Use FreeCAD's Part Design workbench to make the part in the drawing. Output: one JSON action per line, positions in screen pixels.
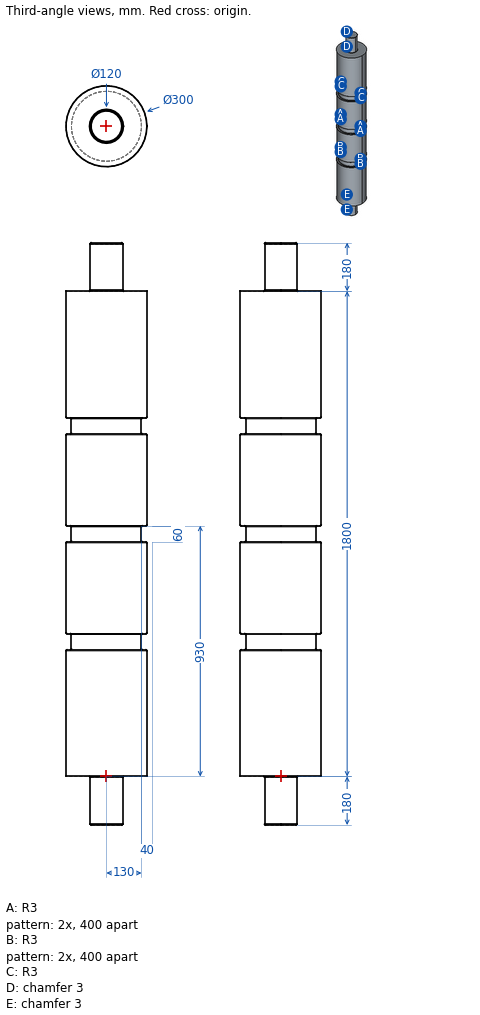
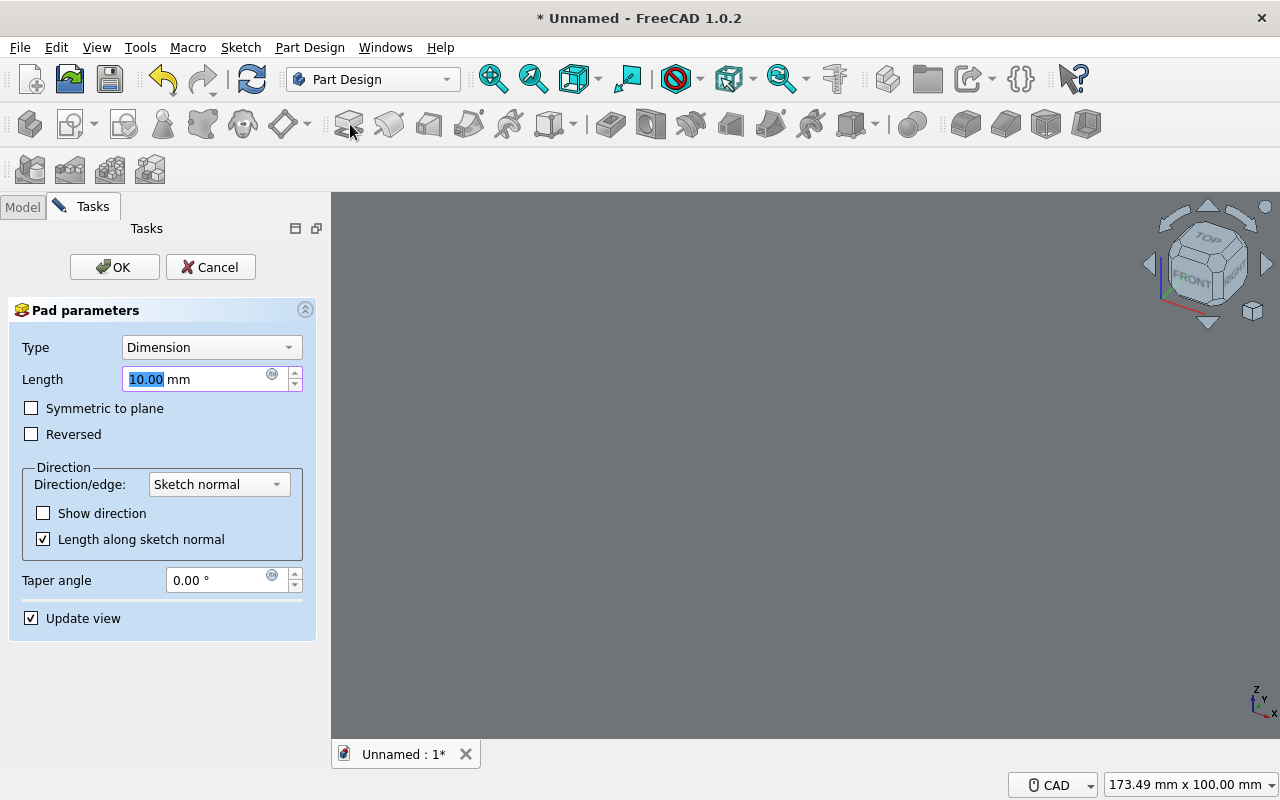
{"action": "type", "text": "1800"}
{"action": "key", "text": "Tab"}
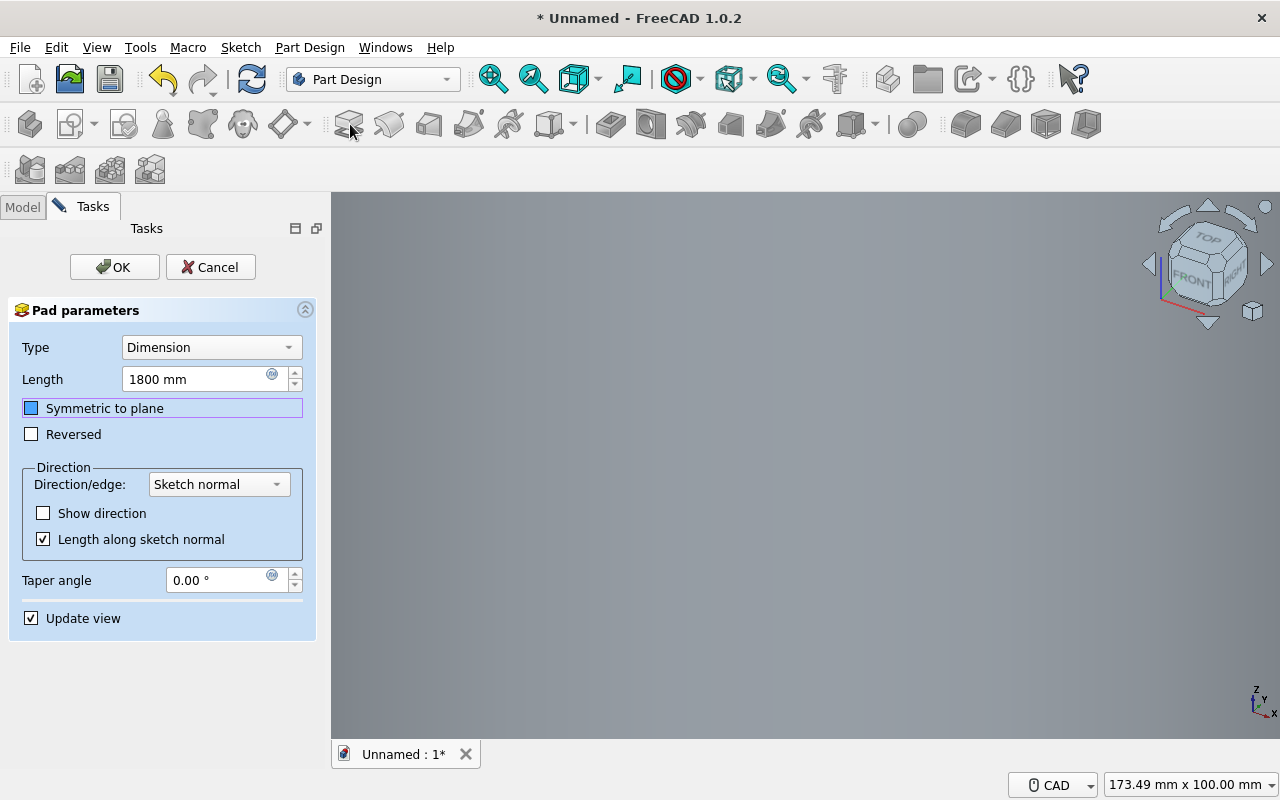
{"action": "left_click", "coordinate": [115, 267]}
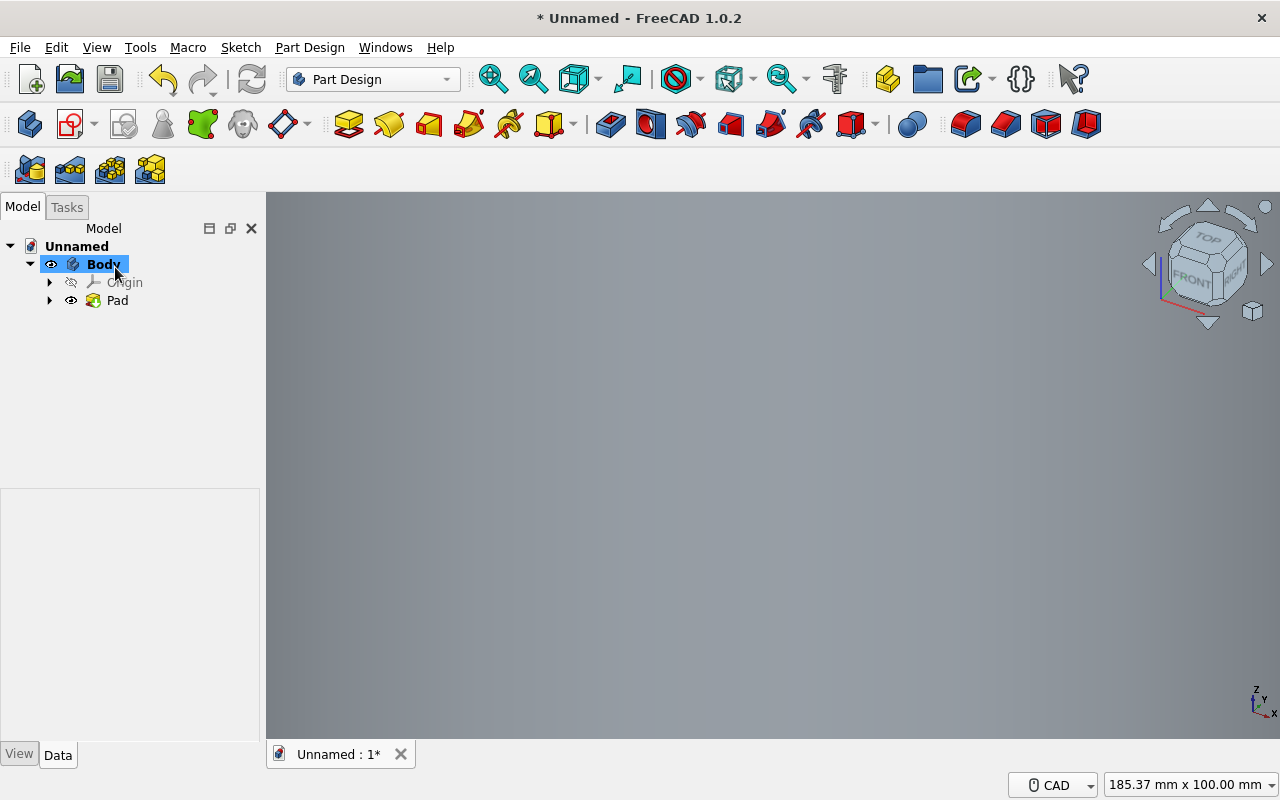
{"action": "left_click", "coordinate": [494, 80]}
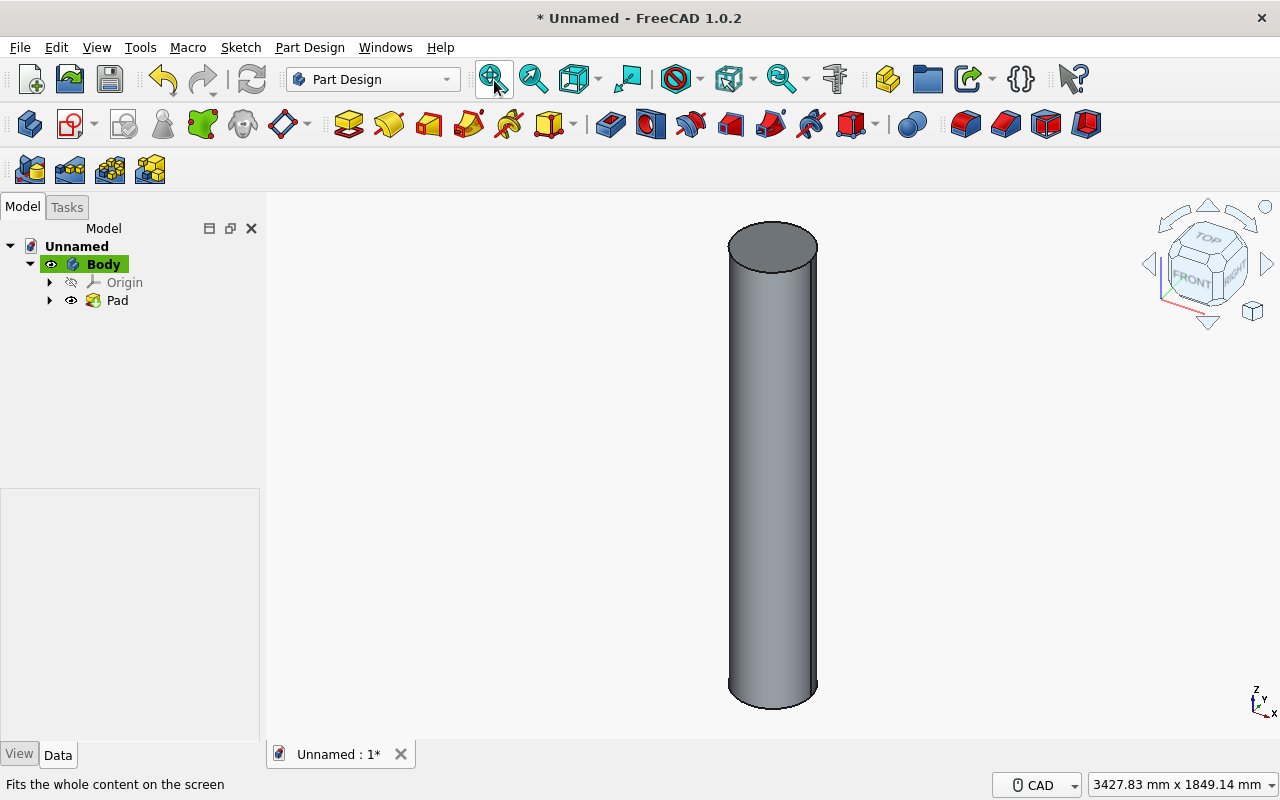
{"action": "left_click", "coordinate": [70, 124]}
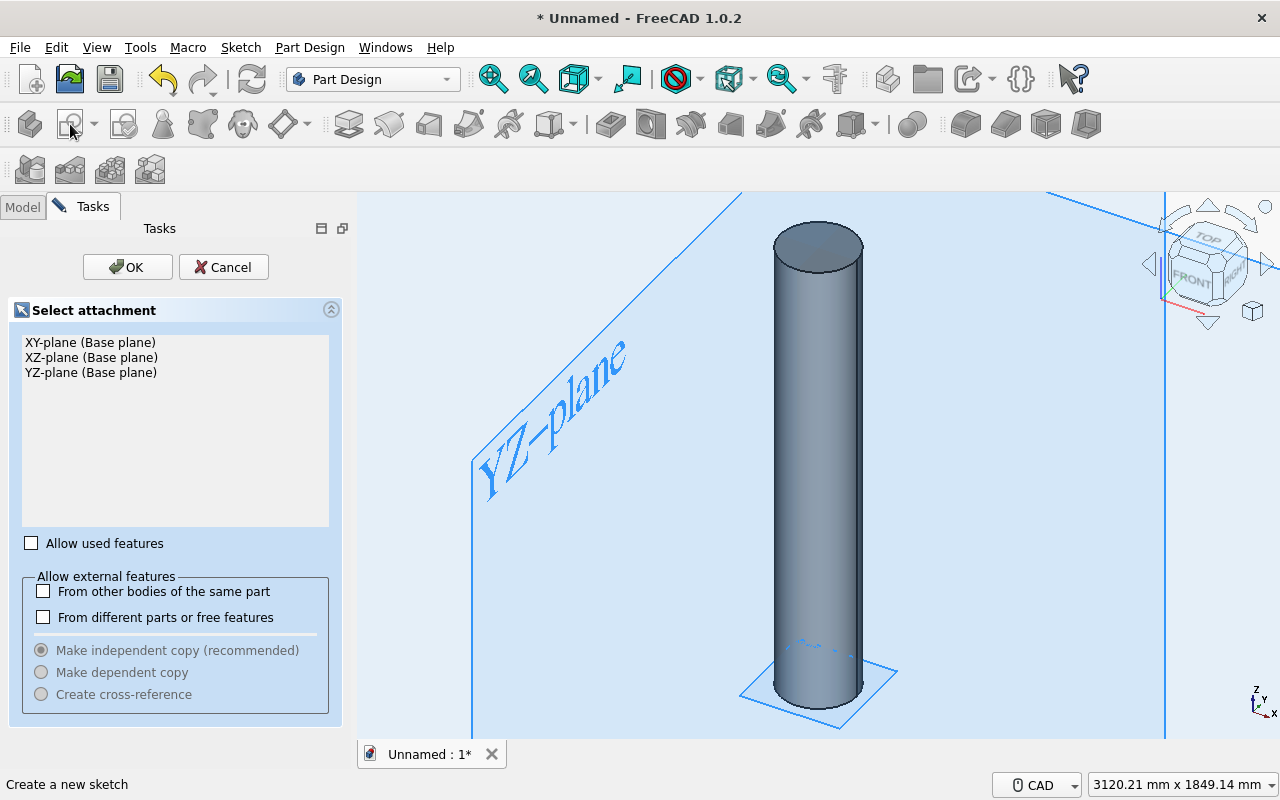
{"action": "left_click", "coordinate": [82, 358]}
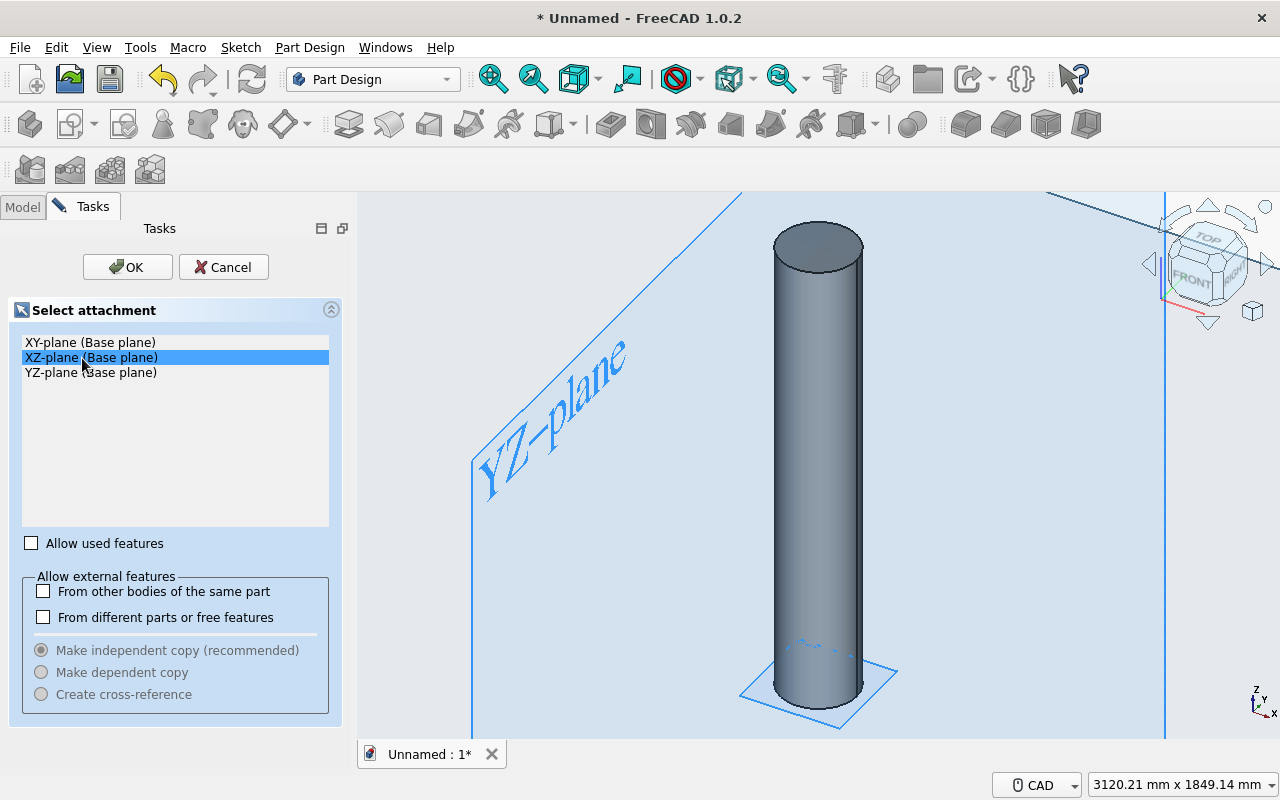
{"action": "left_click", "coordinate": [128, 267]}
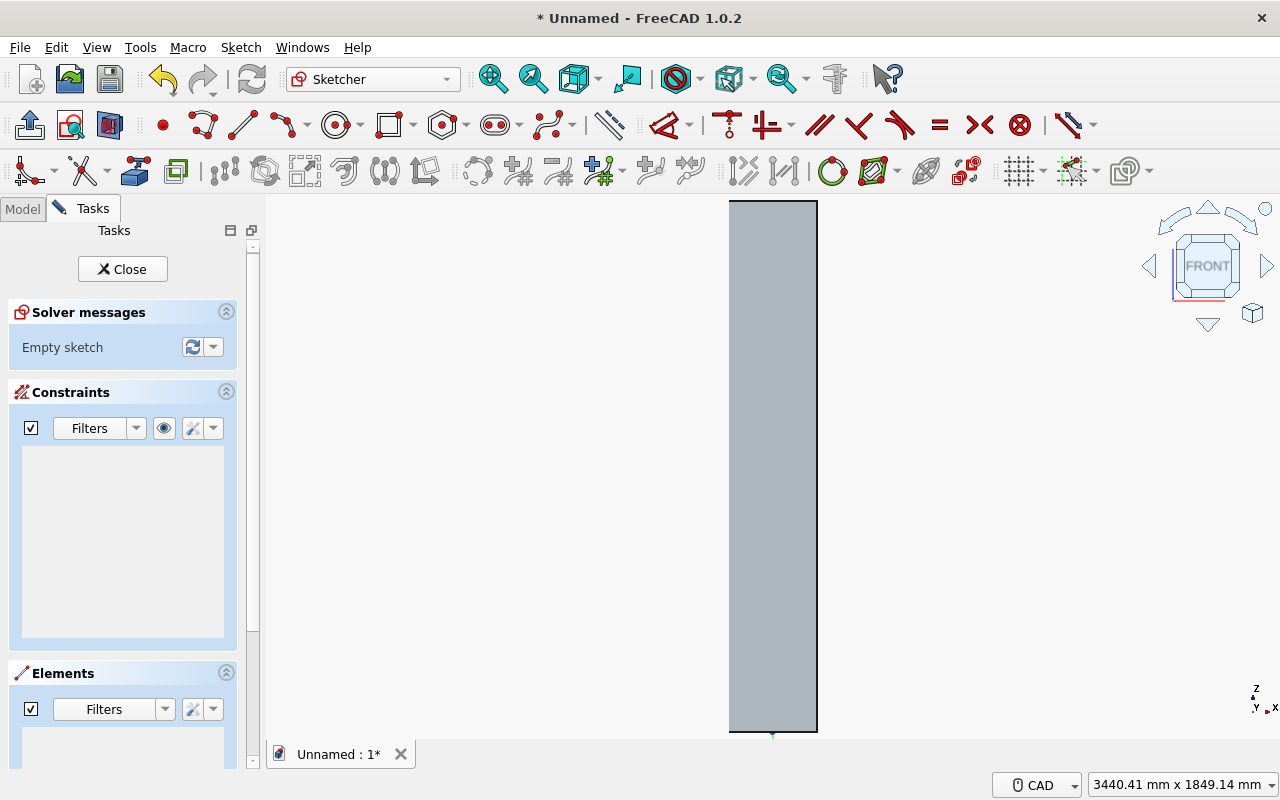
{"action": "left_click", "coordinate": [110, 126]}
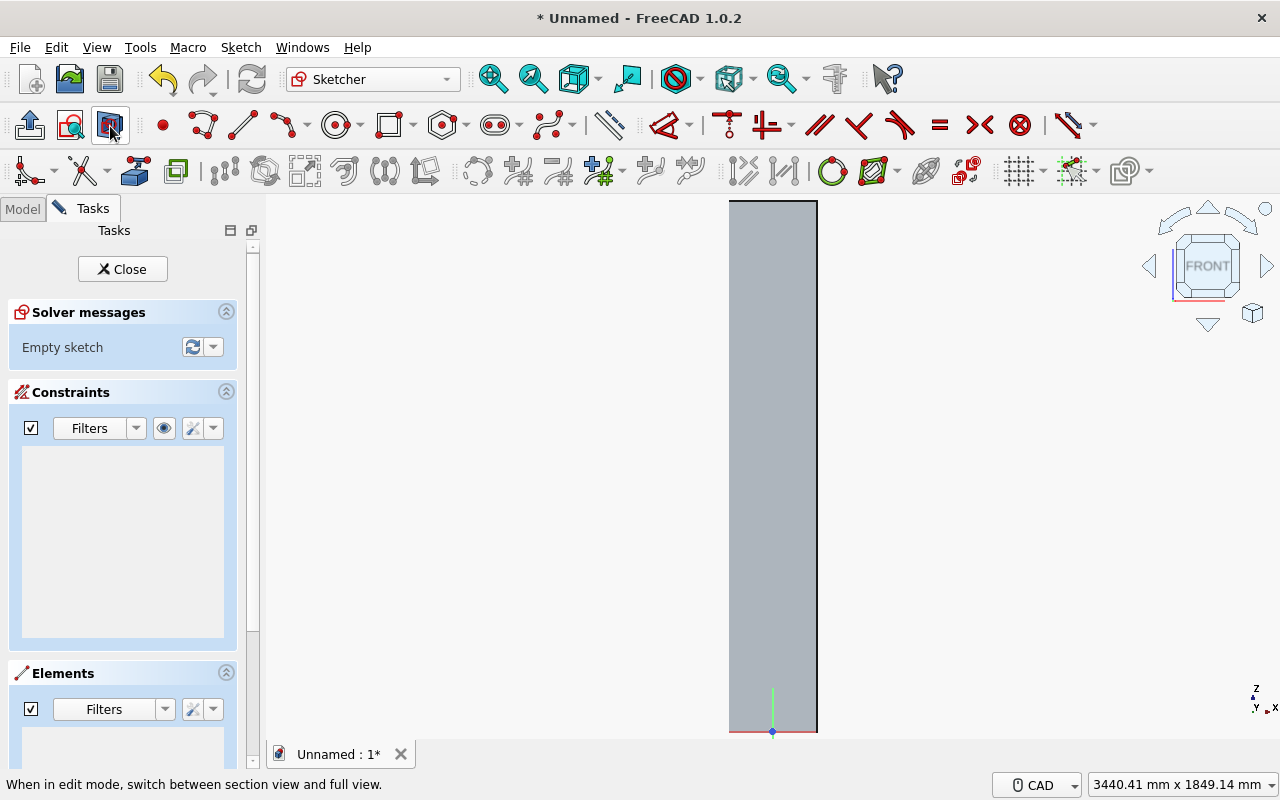
{"action": "scroll", "coordinate": [823, 467], "scroll_direction": "up", "scroll_amount": 15}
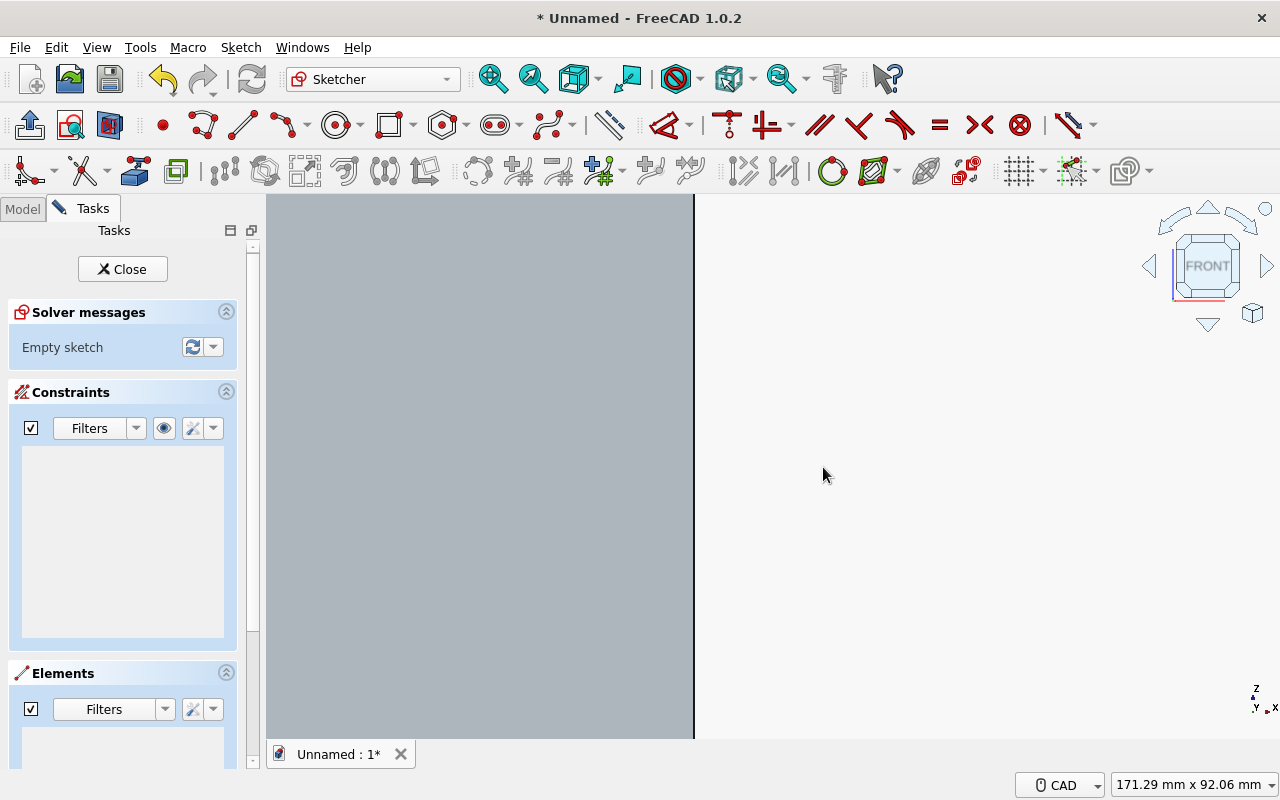
{"action": "left_click", "coordinate": [390, 126]}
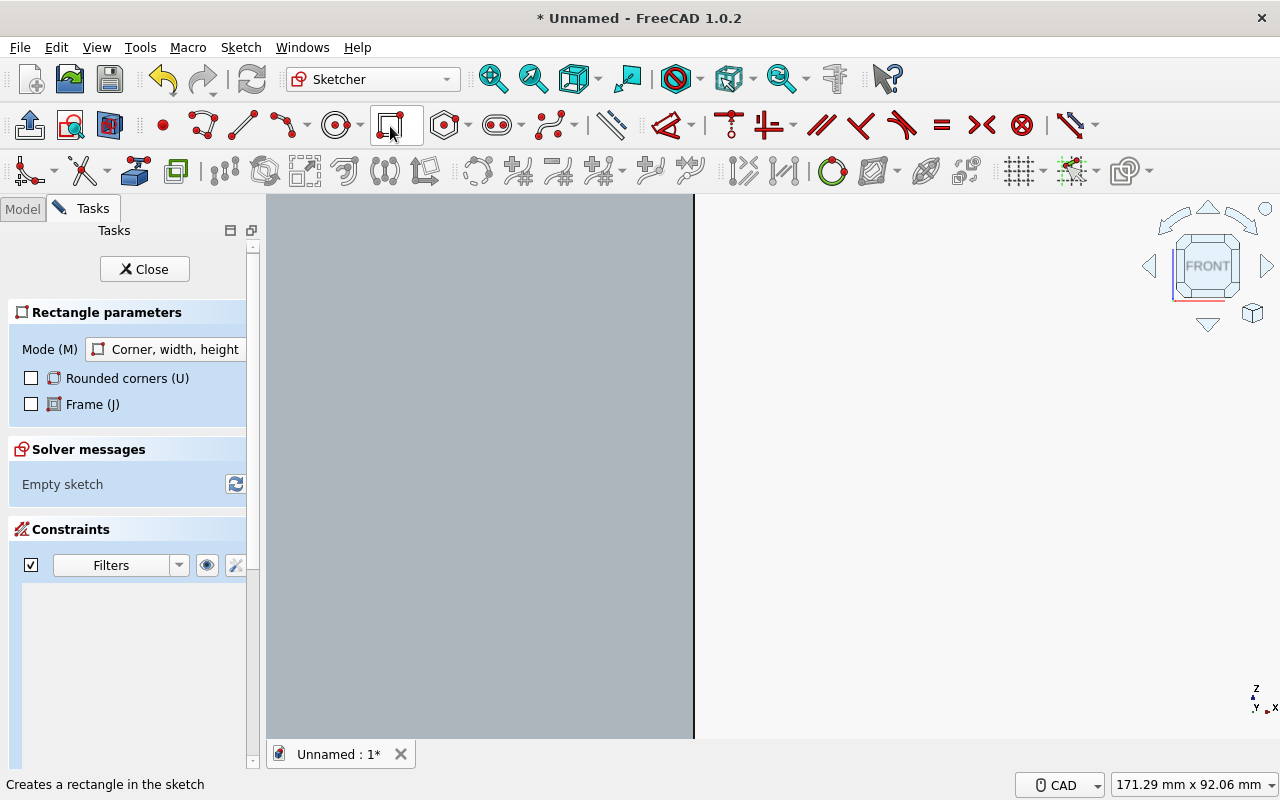
{"action": "left_click", "coordinate": [576, 270]}
{"action": "mouse_move", "coordinate": [812, 625]}